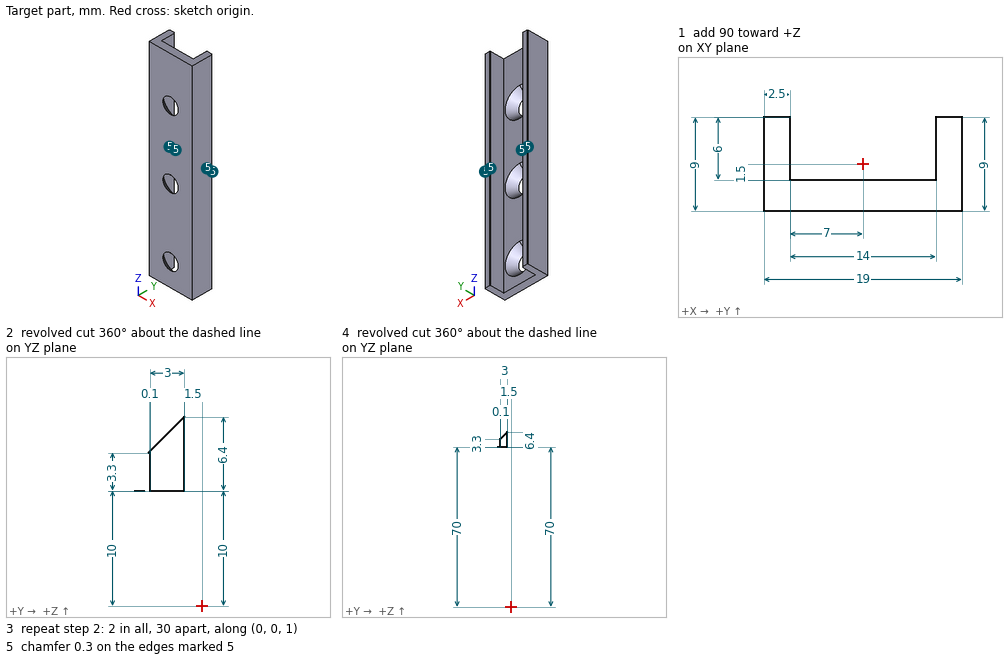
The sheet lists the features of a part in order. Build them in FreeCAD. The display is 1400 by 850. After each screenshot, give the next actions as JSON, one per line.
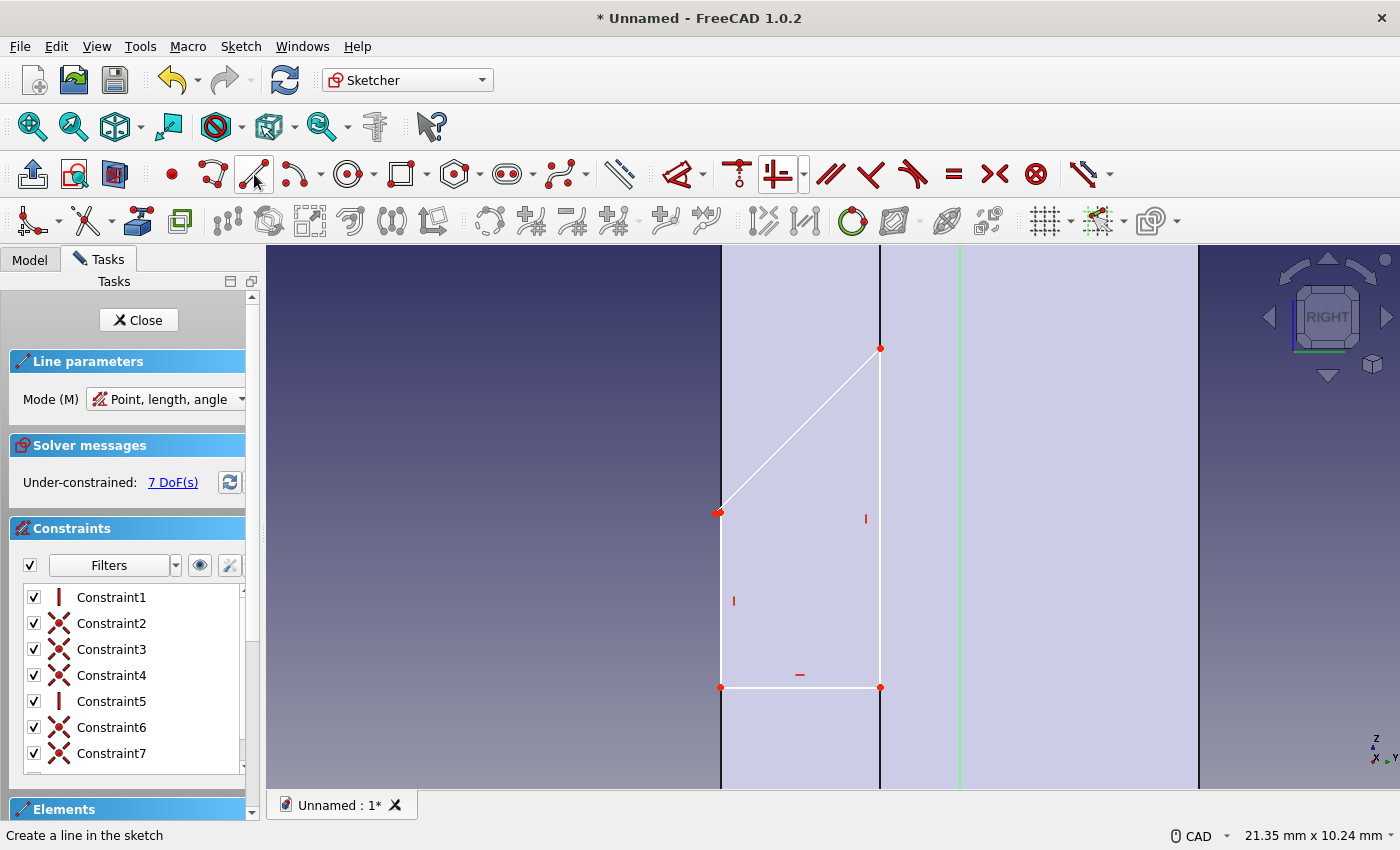
{"action": "left_click", "coordinate": [699, 687]}
{"action": "left_click", "coordinate": [650, 687]}
{"action": "key", "text": "Escape"}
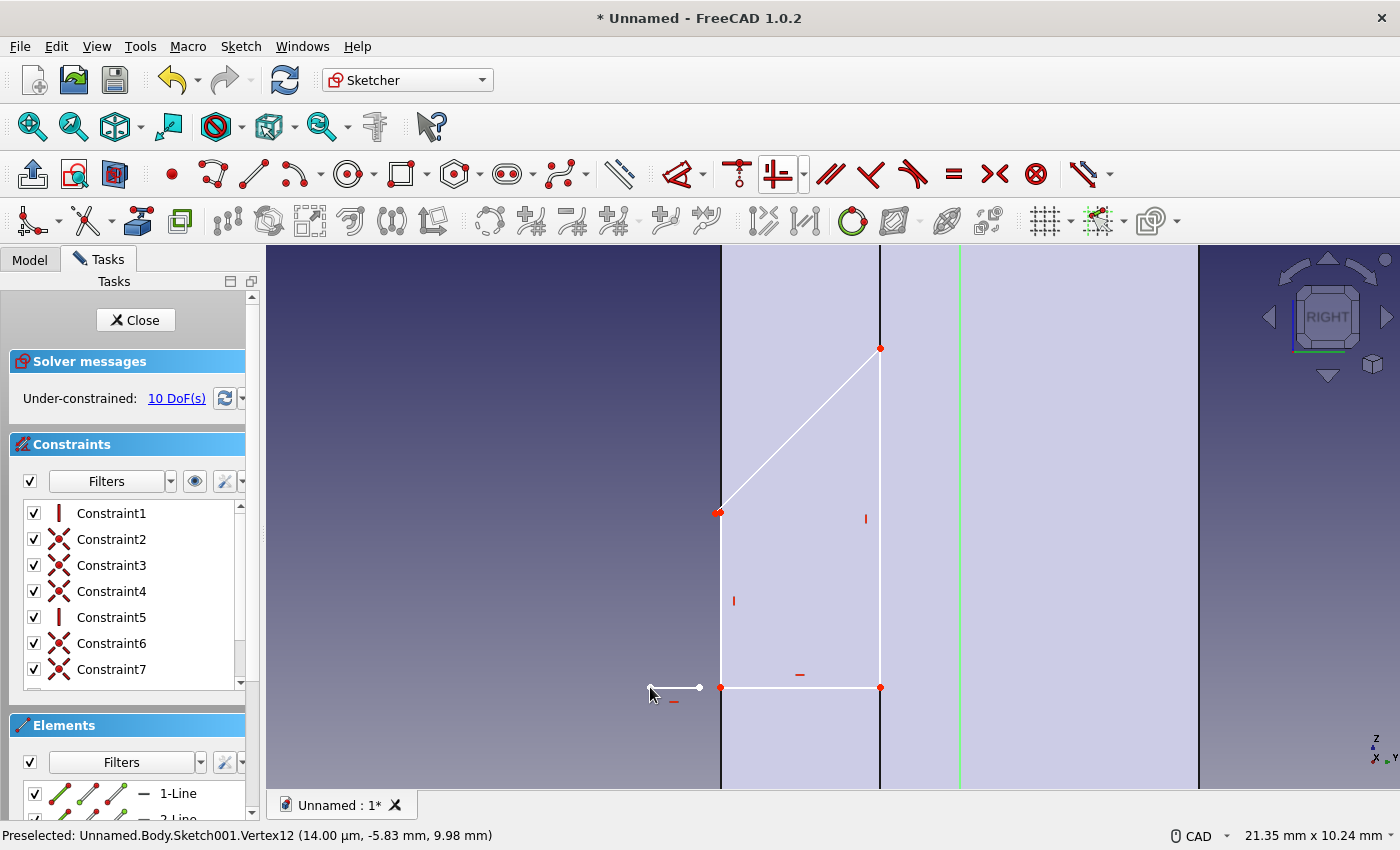
{"action": "left_click", "coordinate": [684, 688]}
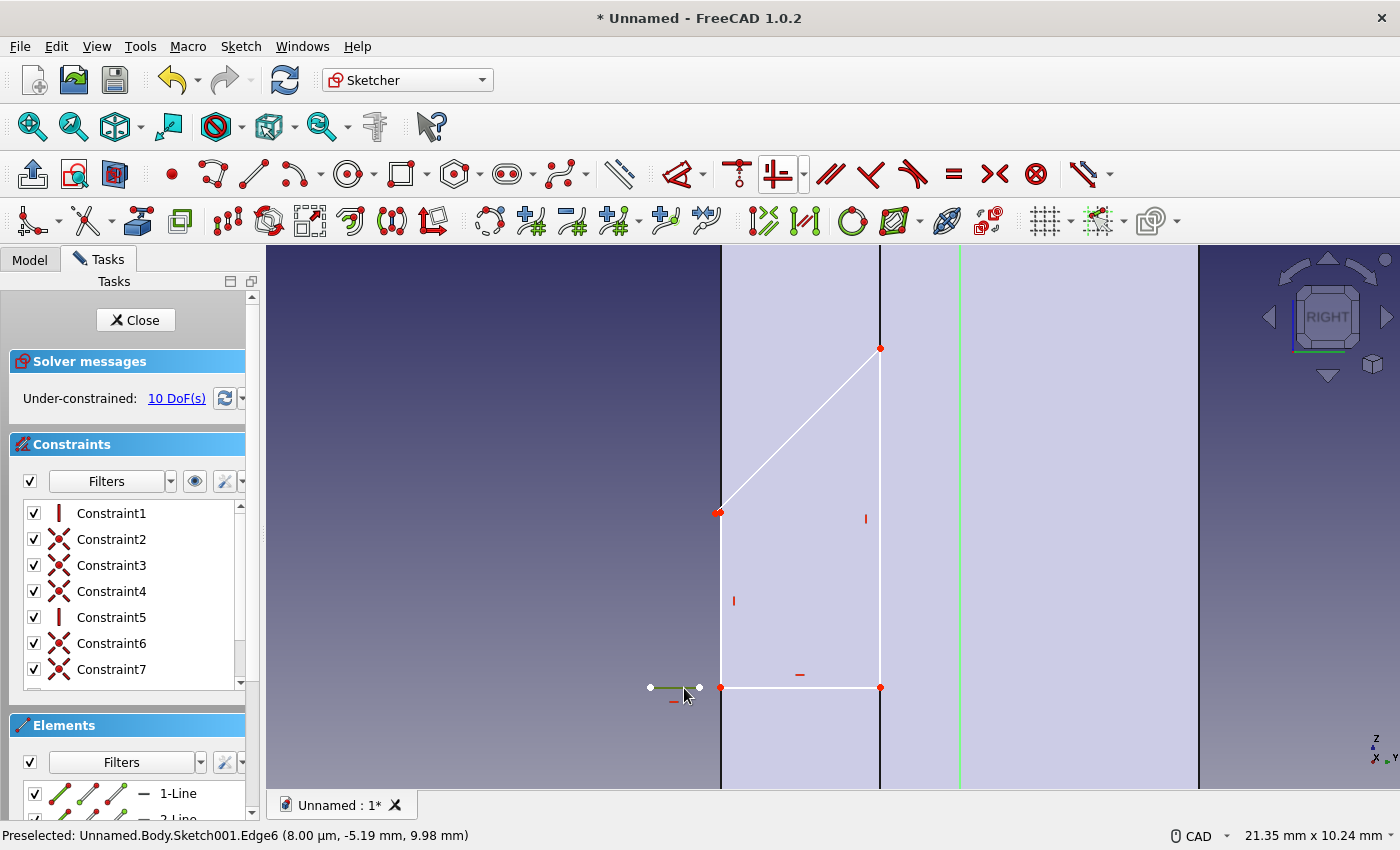
{"action": "left_click", "coordinate": [620, 174]}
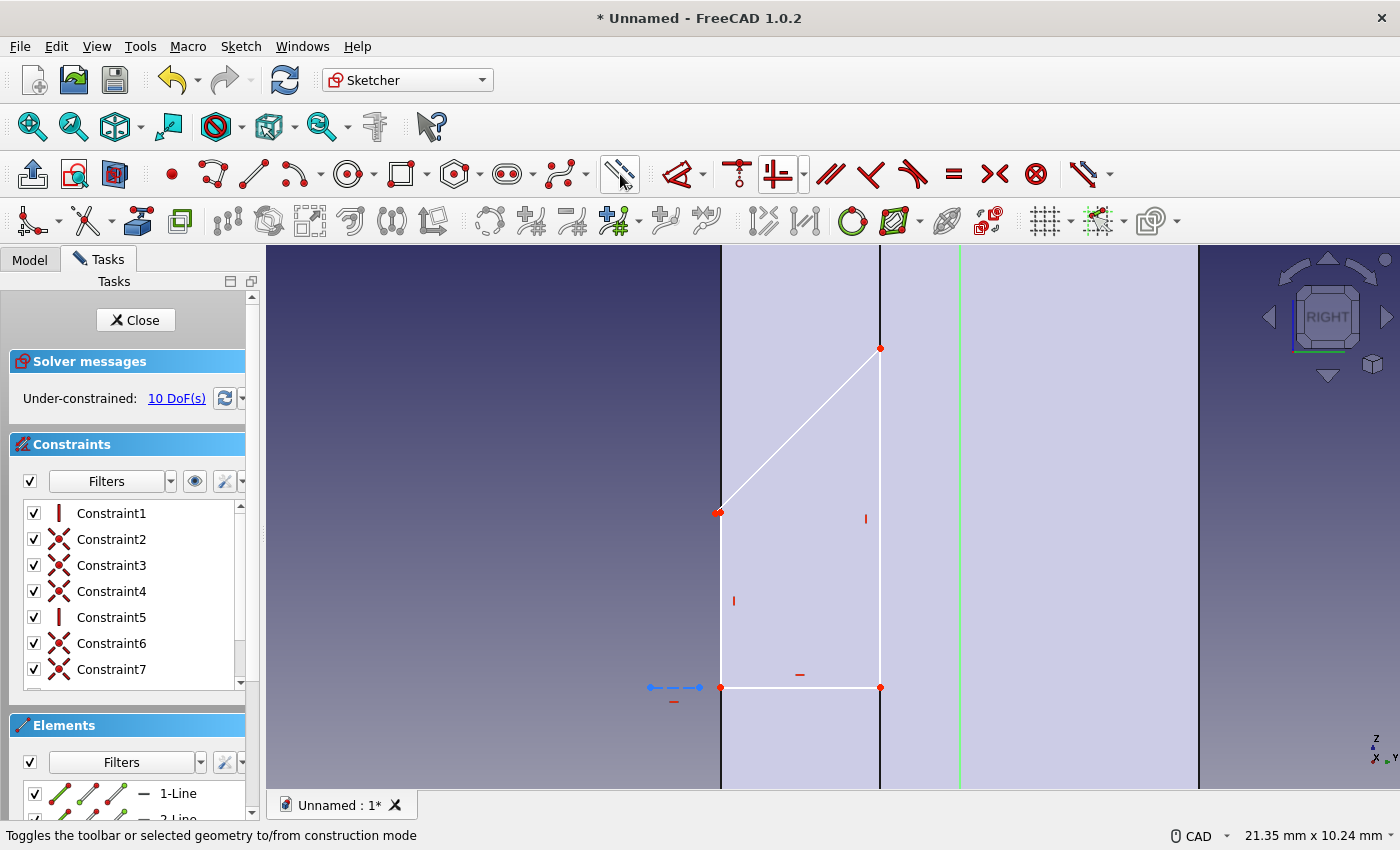
{"action": "scroll", "coordinate": [719, 513], "scroll_direction": "up", "scroll_amount": 10}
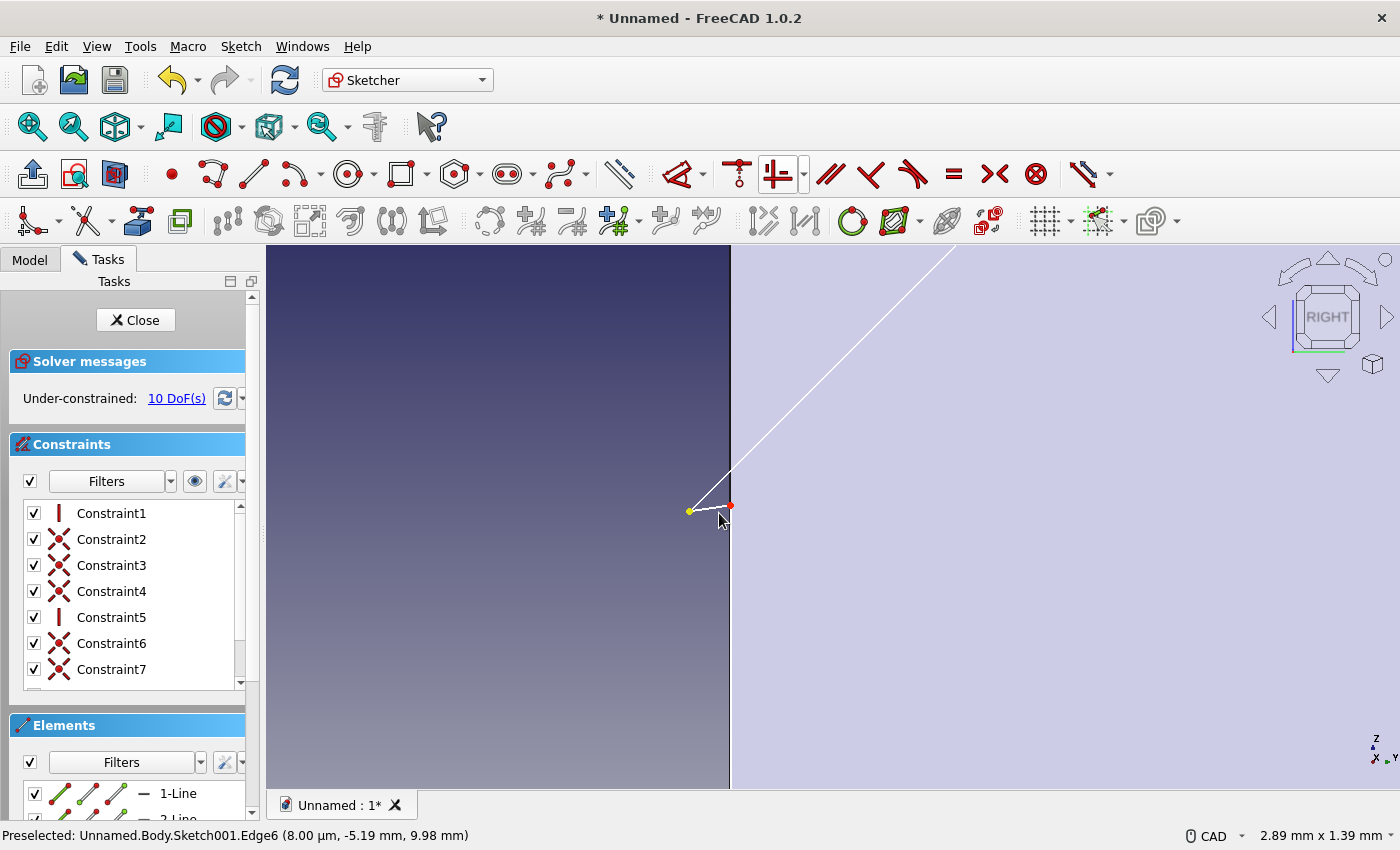
{"action": "left_click", "coordinate": [714, 508]}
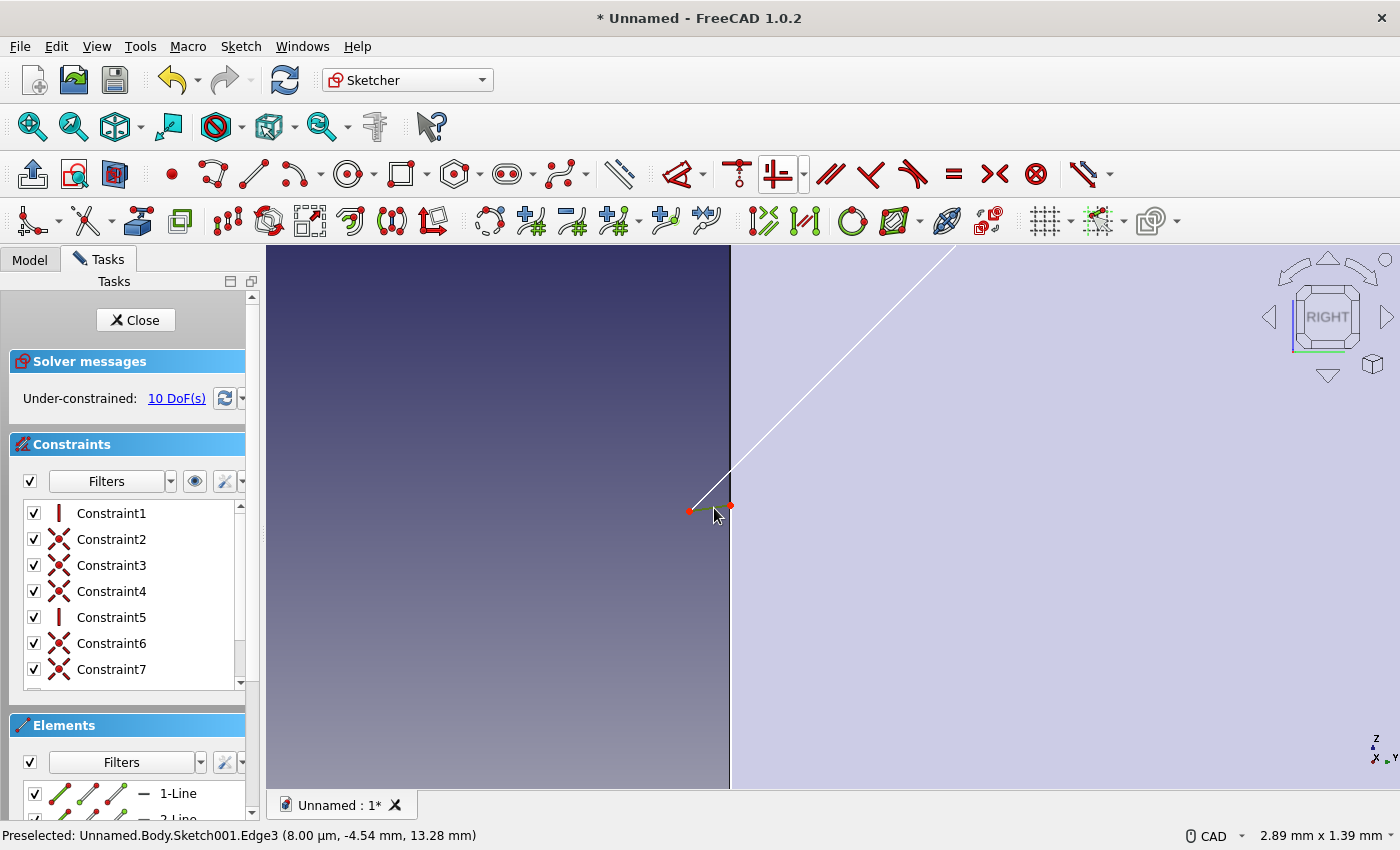
{"action": "left_click", "coordinate": [804, 174]}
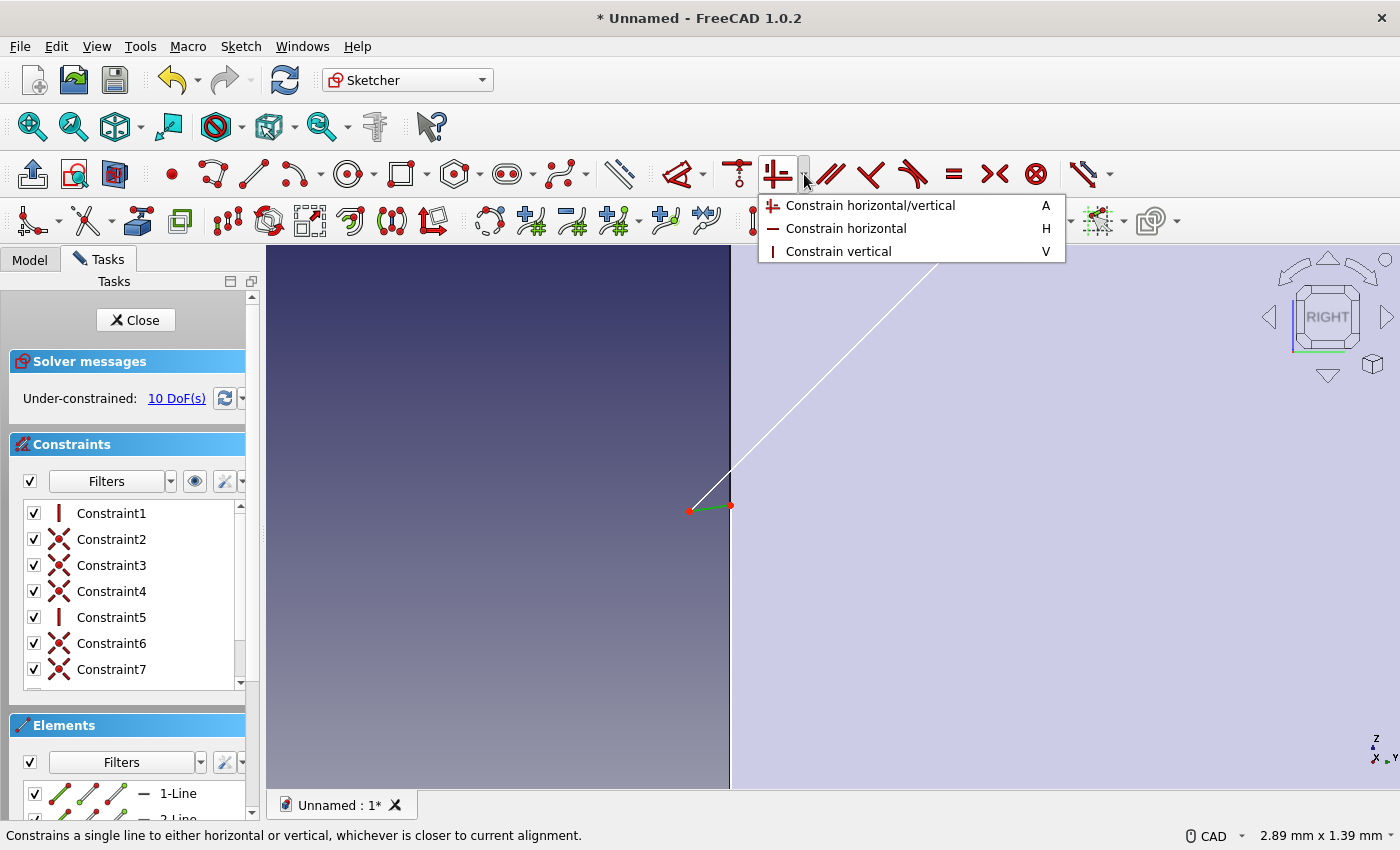
{"action": "left_click", "coordinate": [912, 228]}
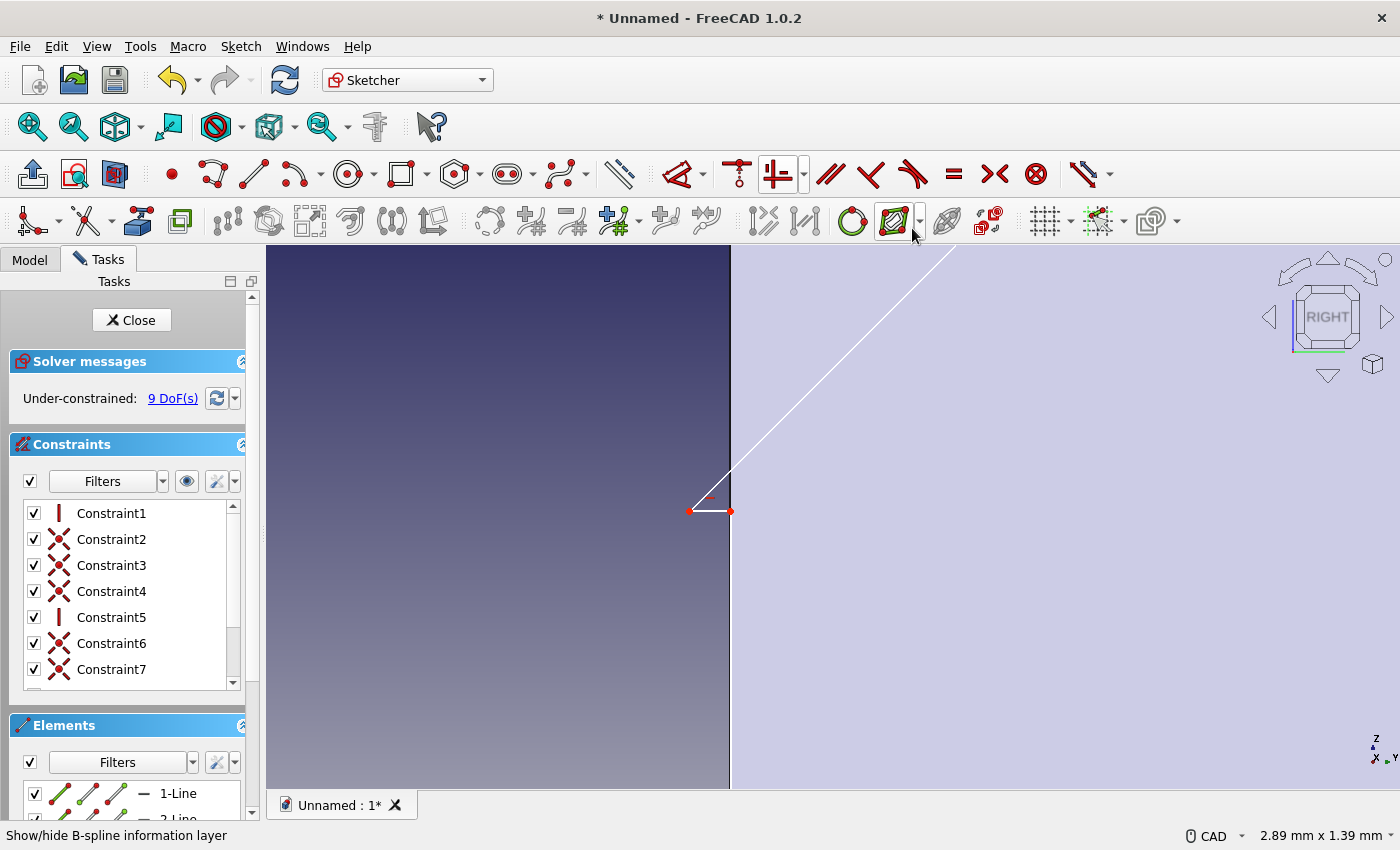
{"action": "left_click", "coordinate": [676, 174]}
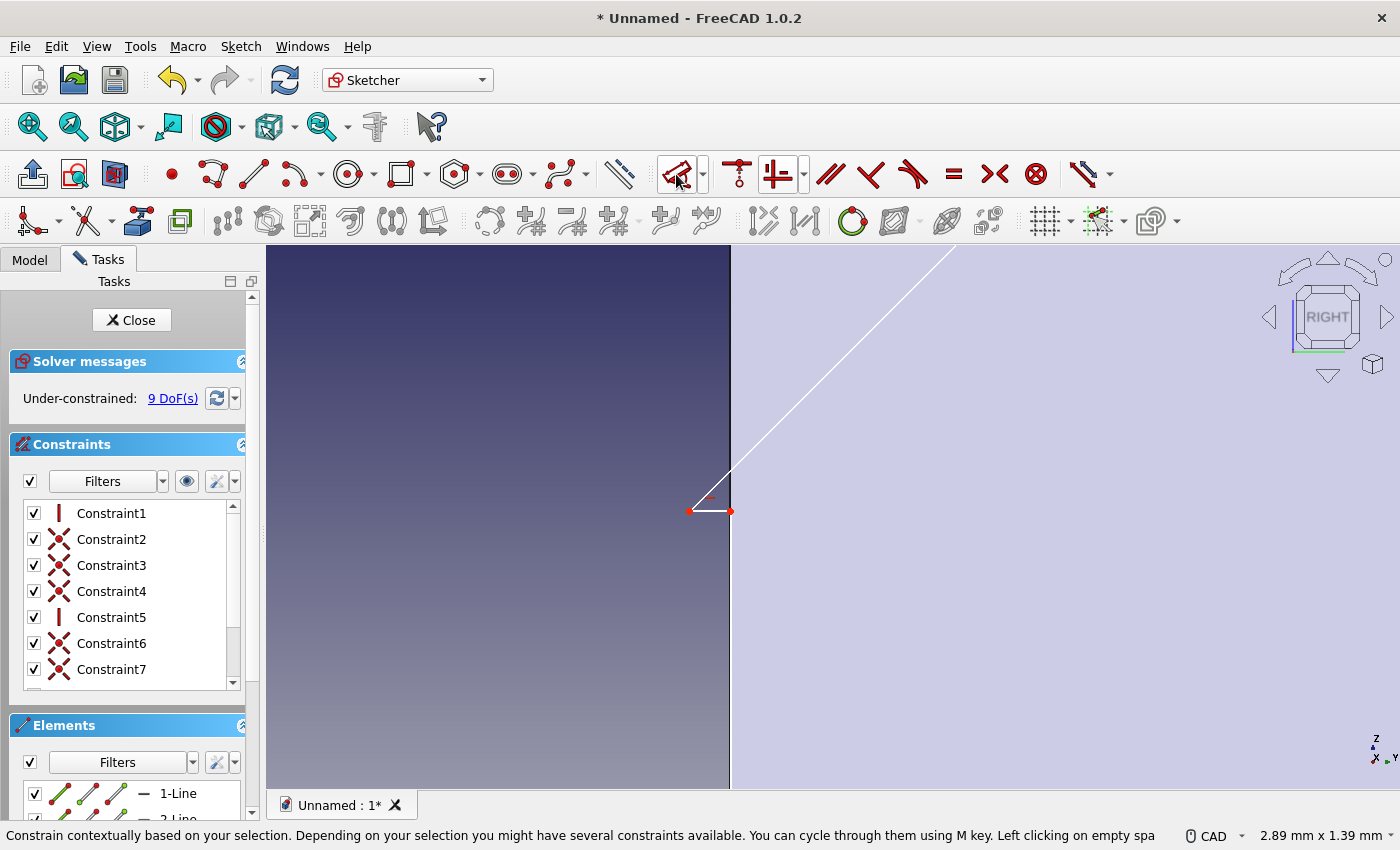
{"action": "scroll", "coordinate": [719, 513], "scroll_direction": "down", "scroll_amount": 10}